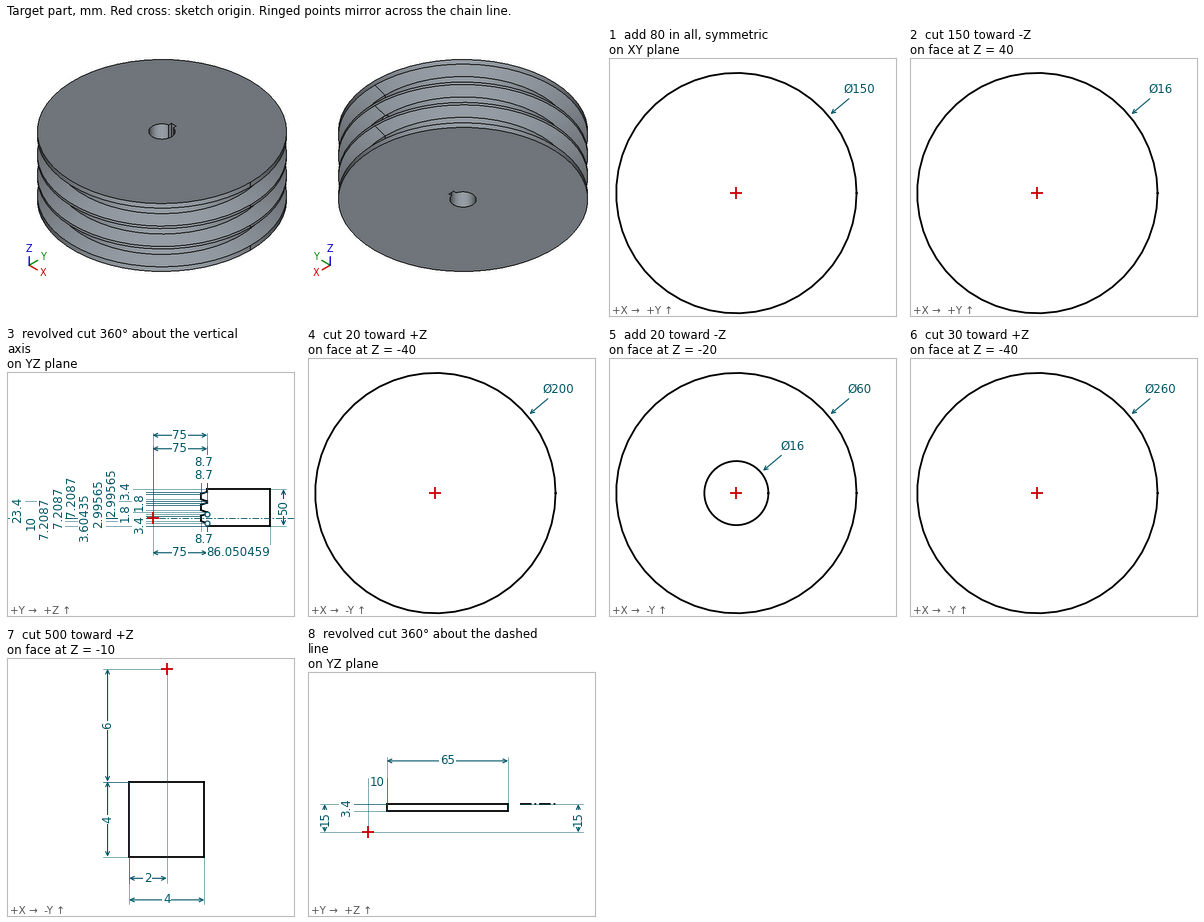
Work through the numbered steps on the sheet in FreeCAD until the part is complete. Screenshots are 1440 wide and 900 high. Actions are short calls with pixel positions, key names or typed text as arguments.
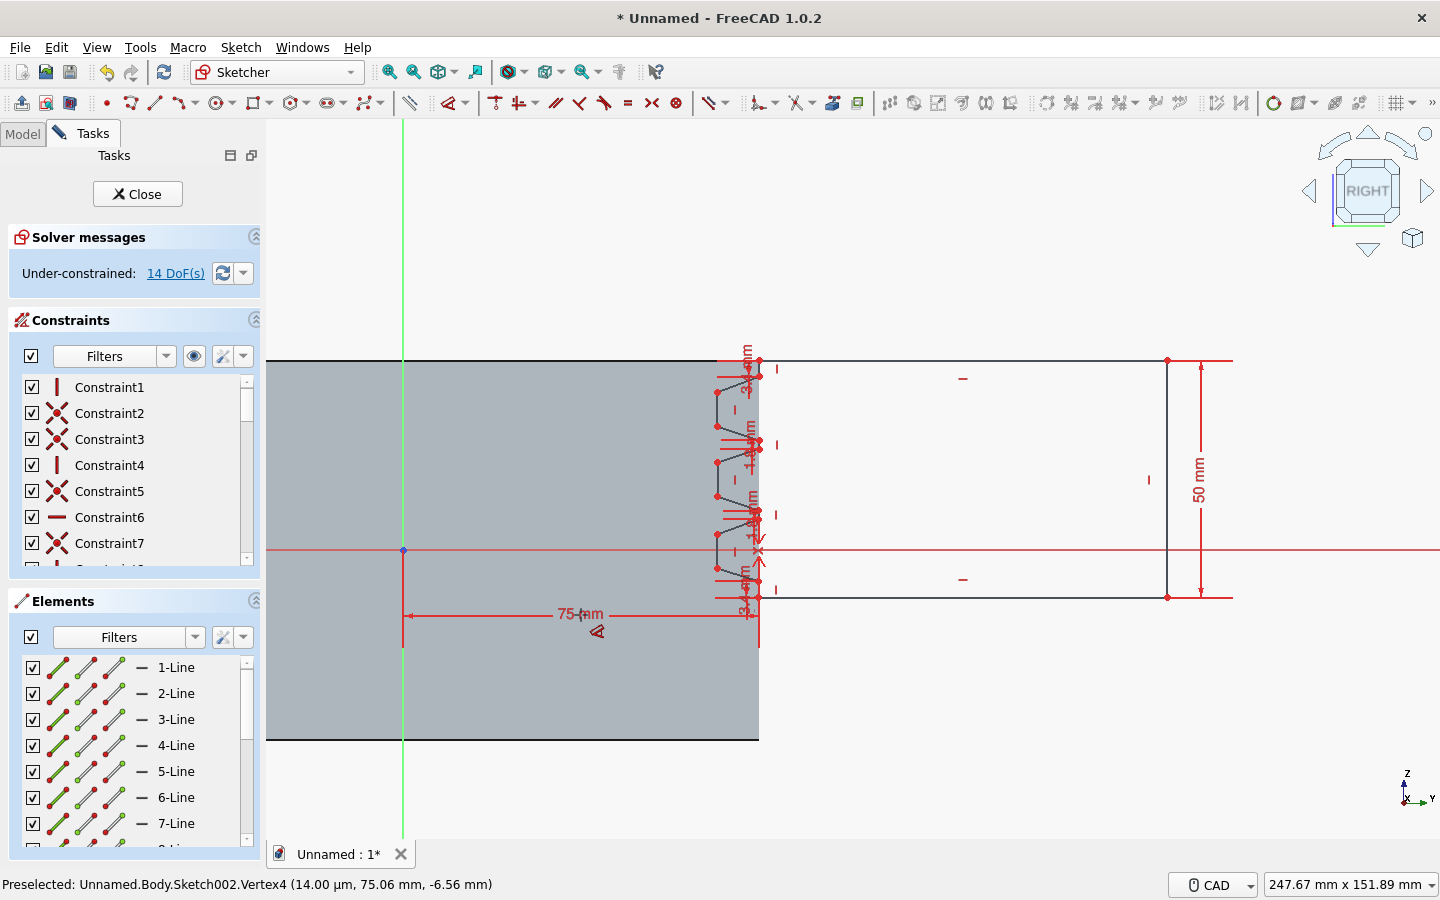
click(759, 598)
click(369, 574)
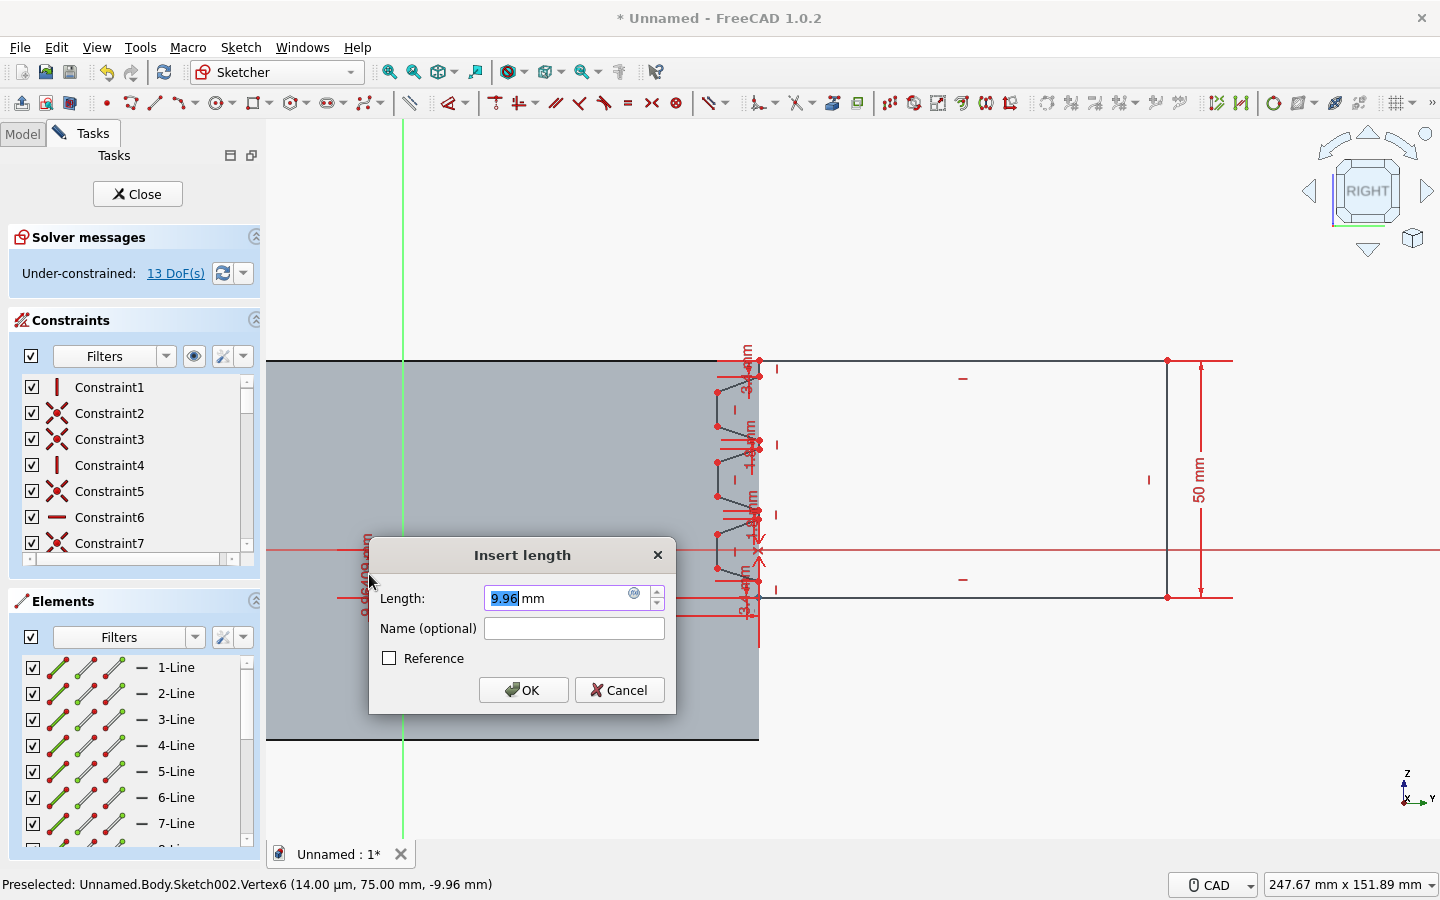
text(10)
key(Return)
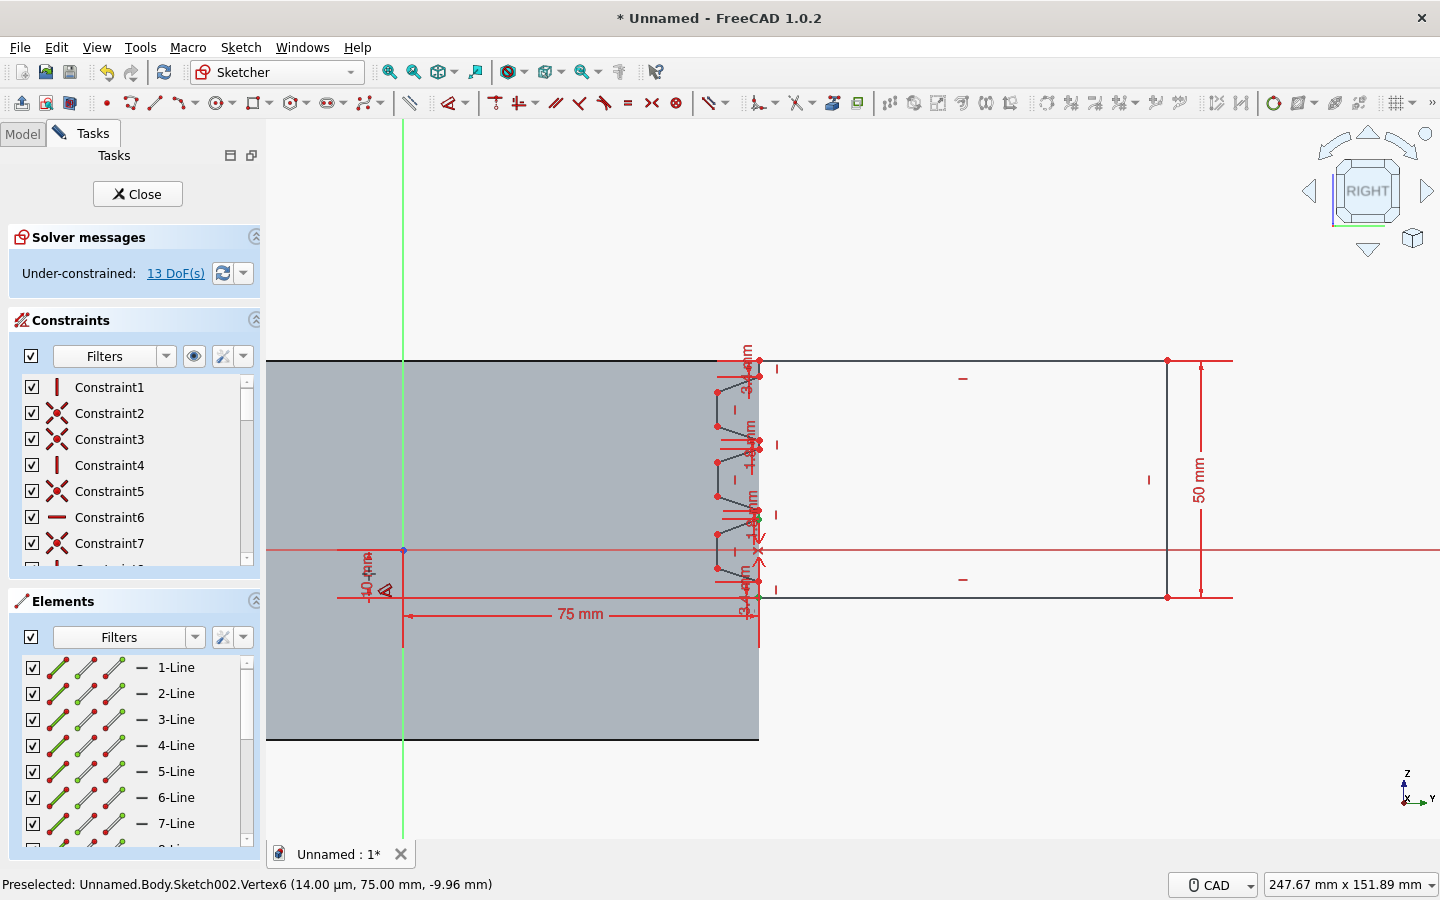
click(759, 361)
click(581, 327)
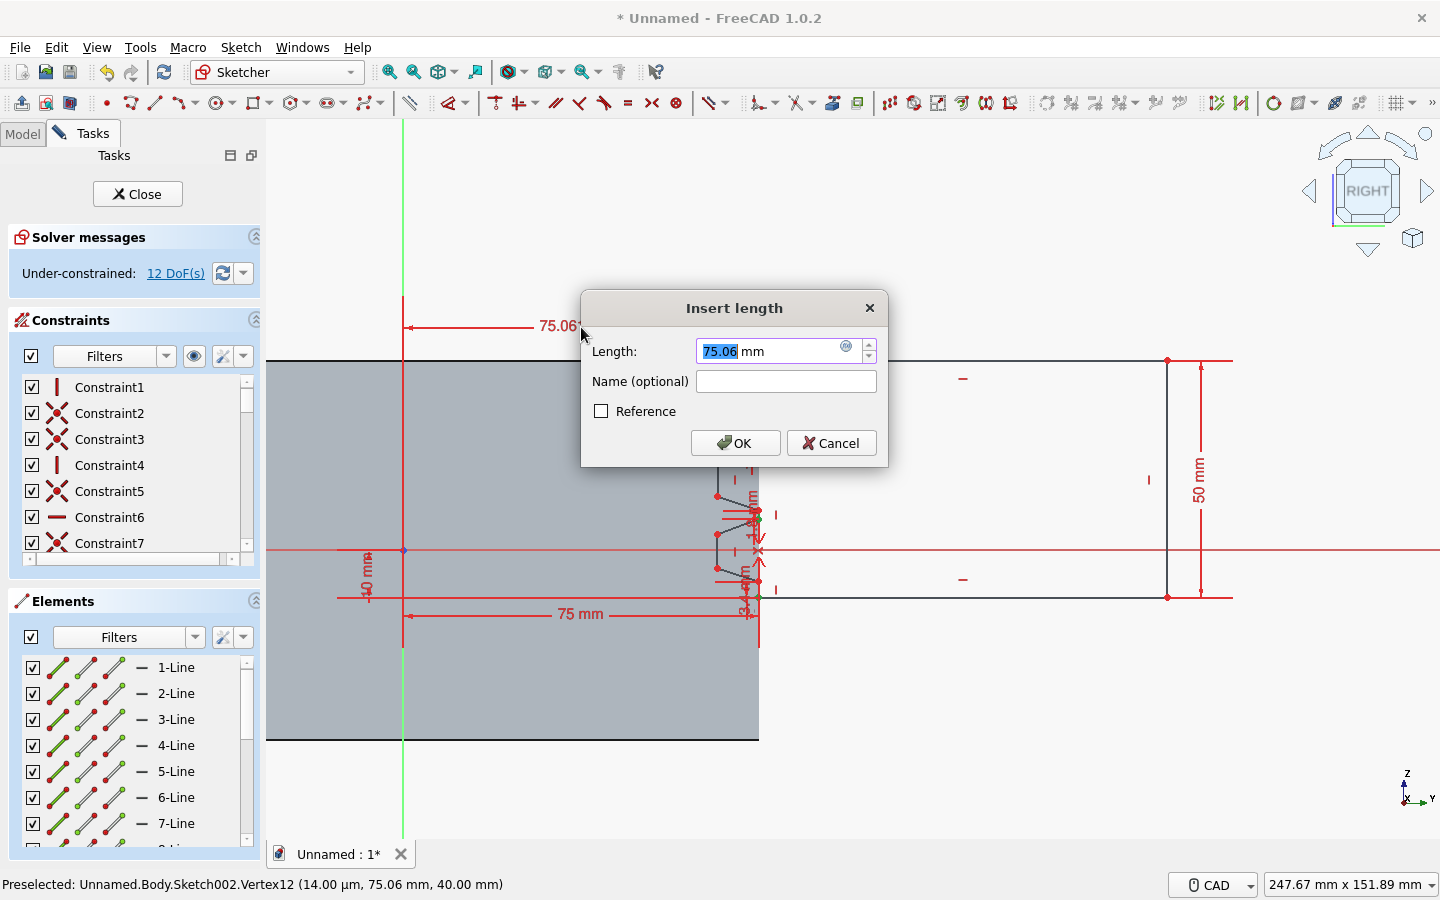
text(75)
key(Return)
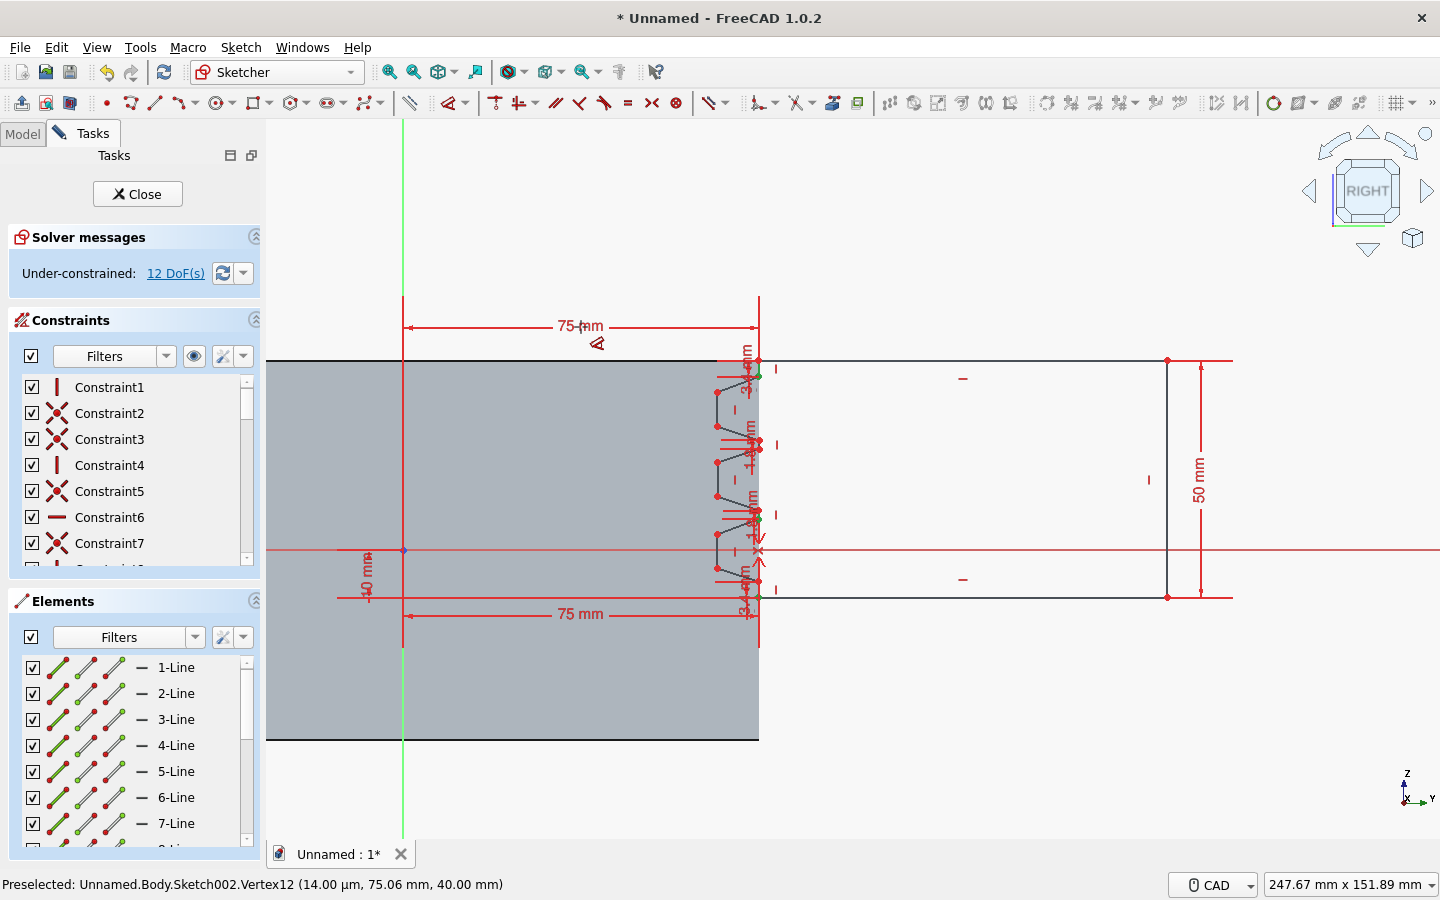
scroll(759, 440, up, 2)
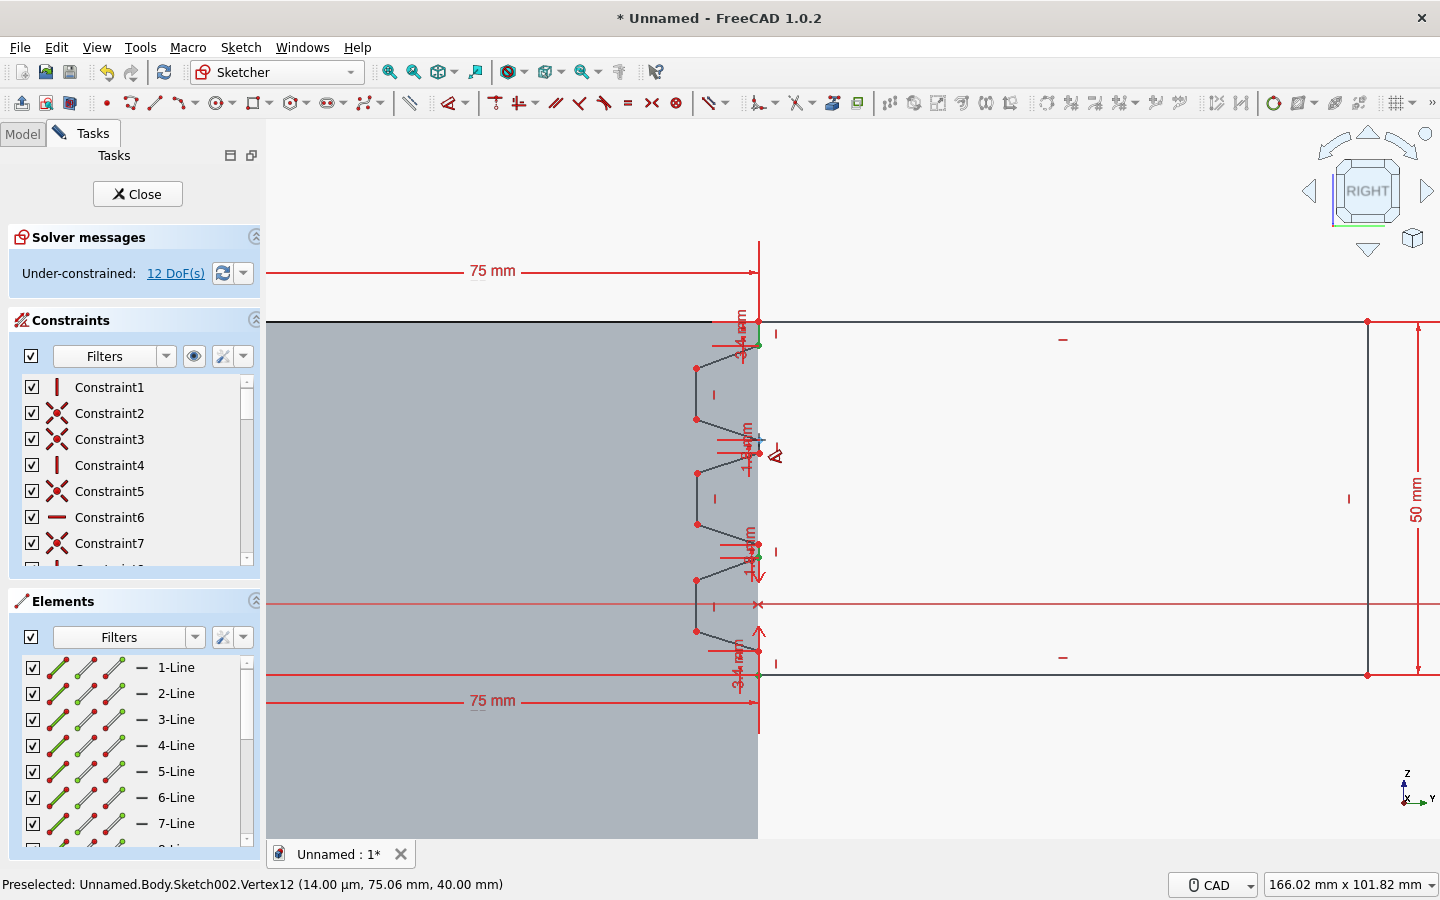
click(759, 440)
click(527, 638)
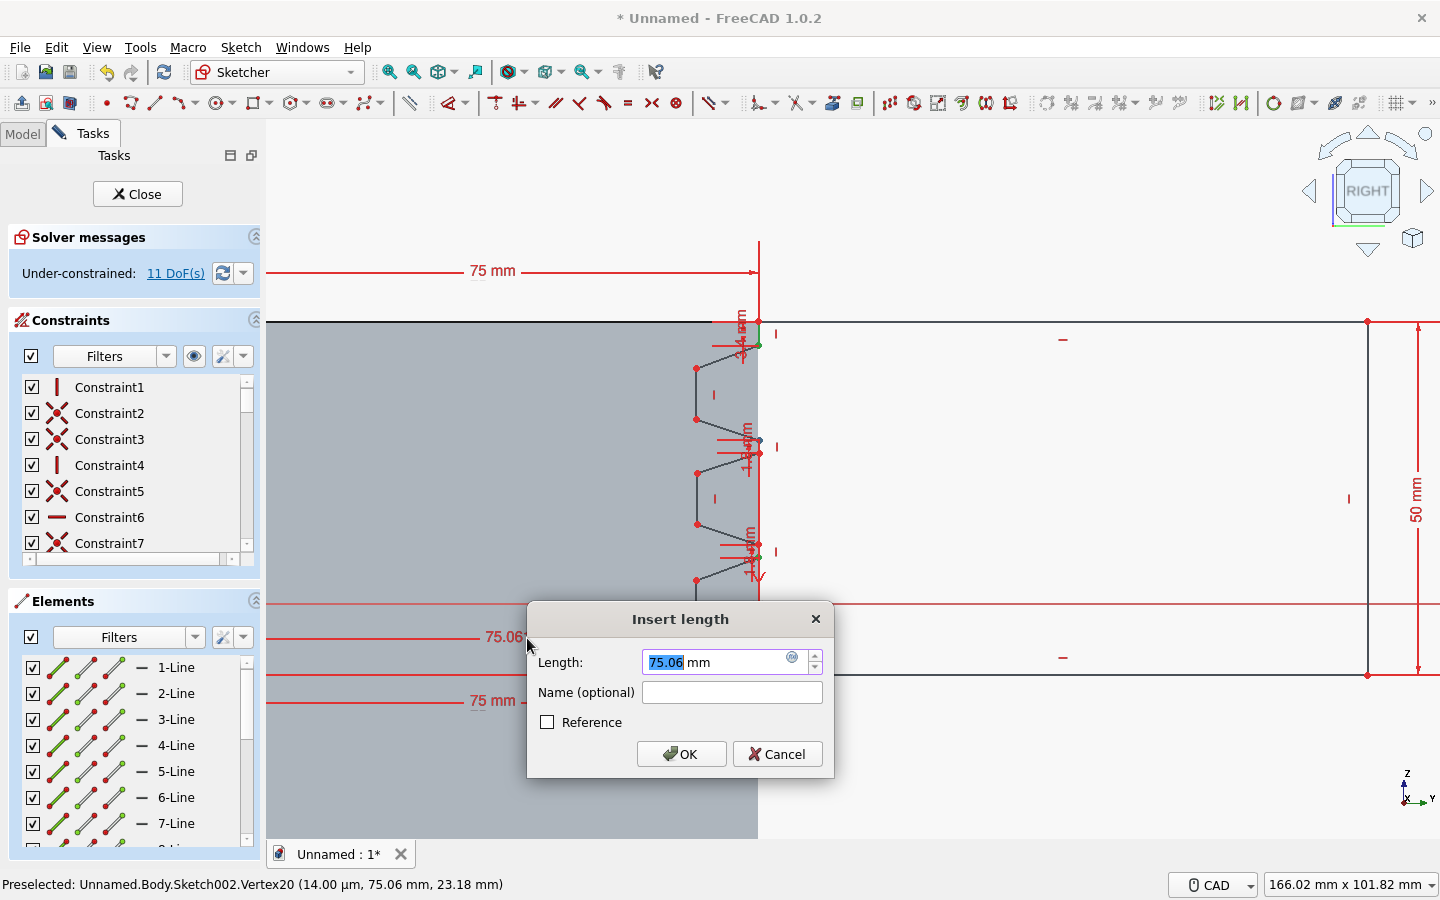
text(75)
key(Return)